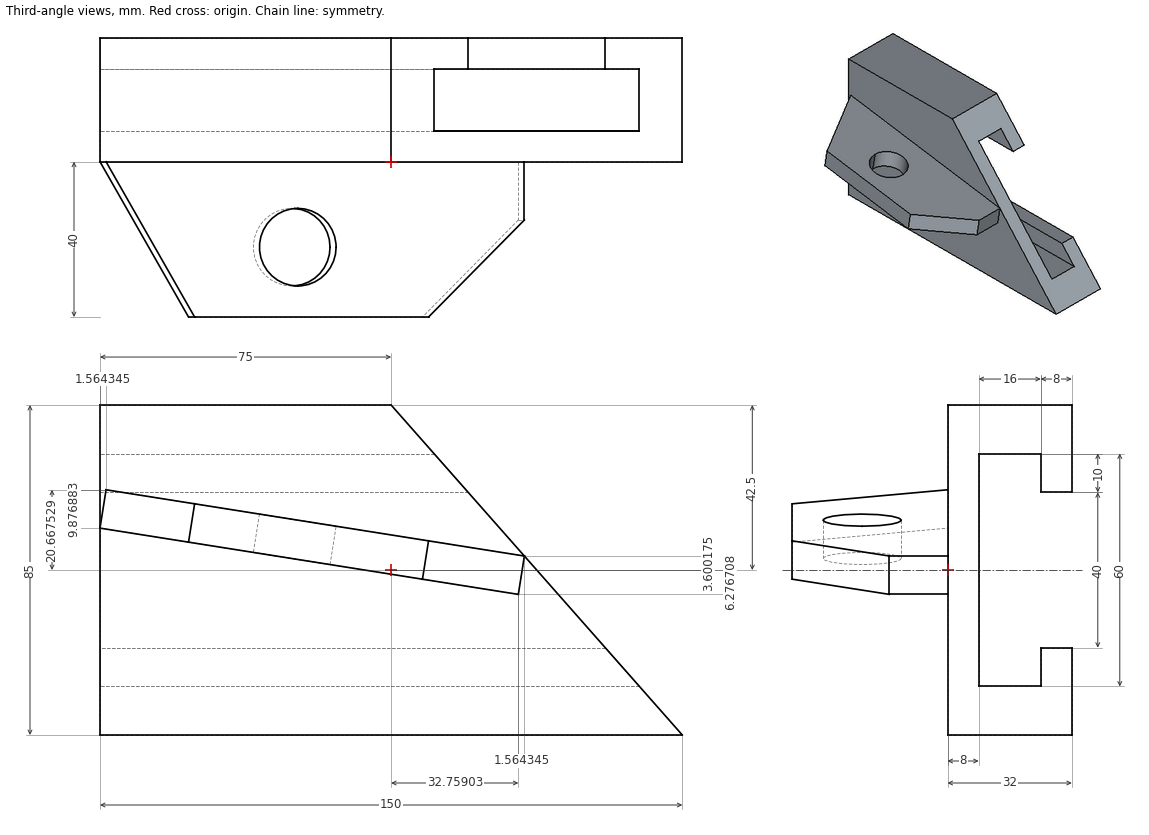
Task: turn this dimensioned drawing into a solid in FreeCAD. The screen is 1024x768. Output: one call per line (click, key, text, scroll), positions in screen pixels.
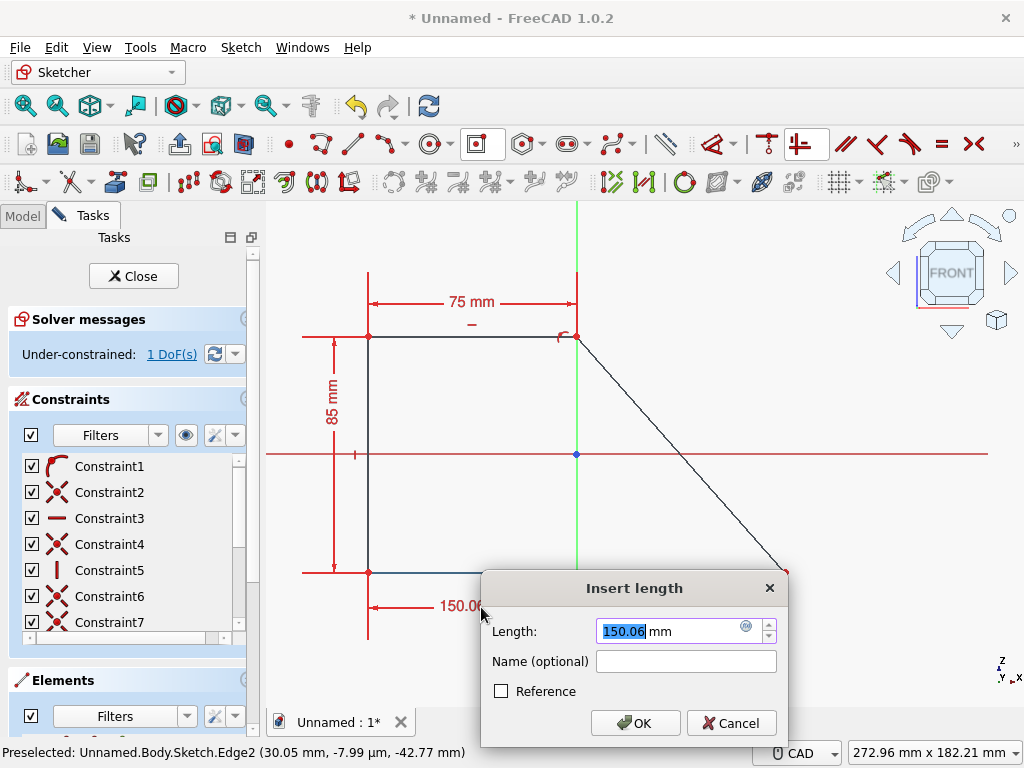
text(150)
key(Return)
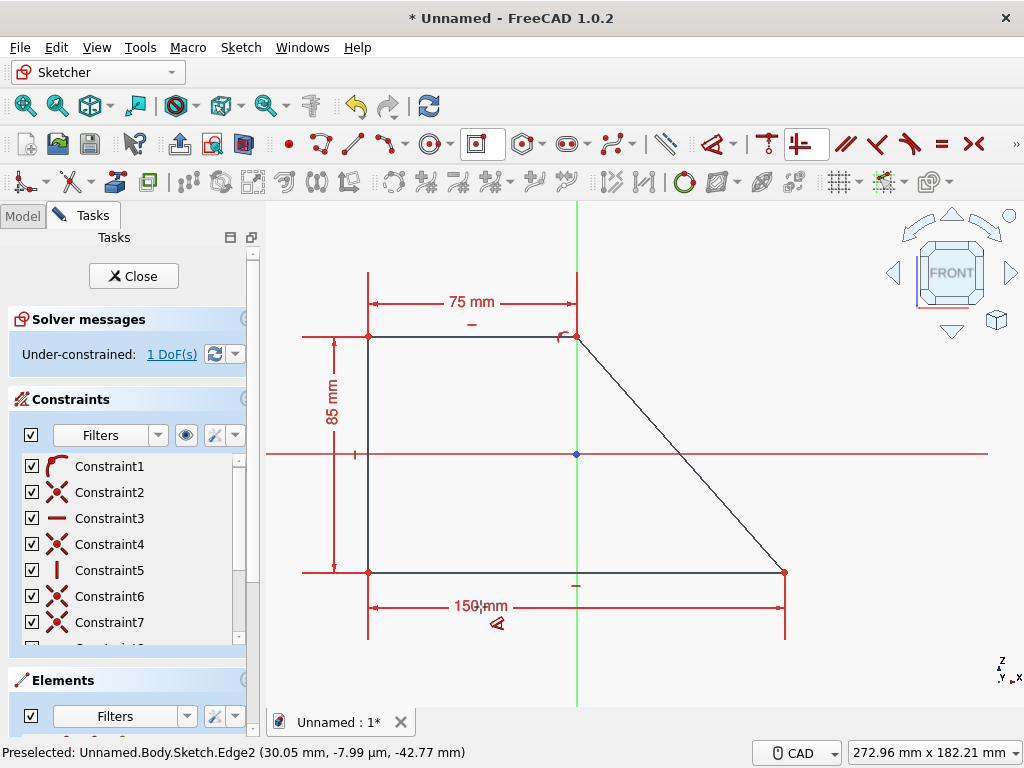
click(577, 337)
click(611, 396)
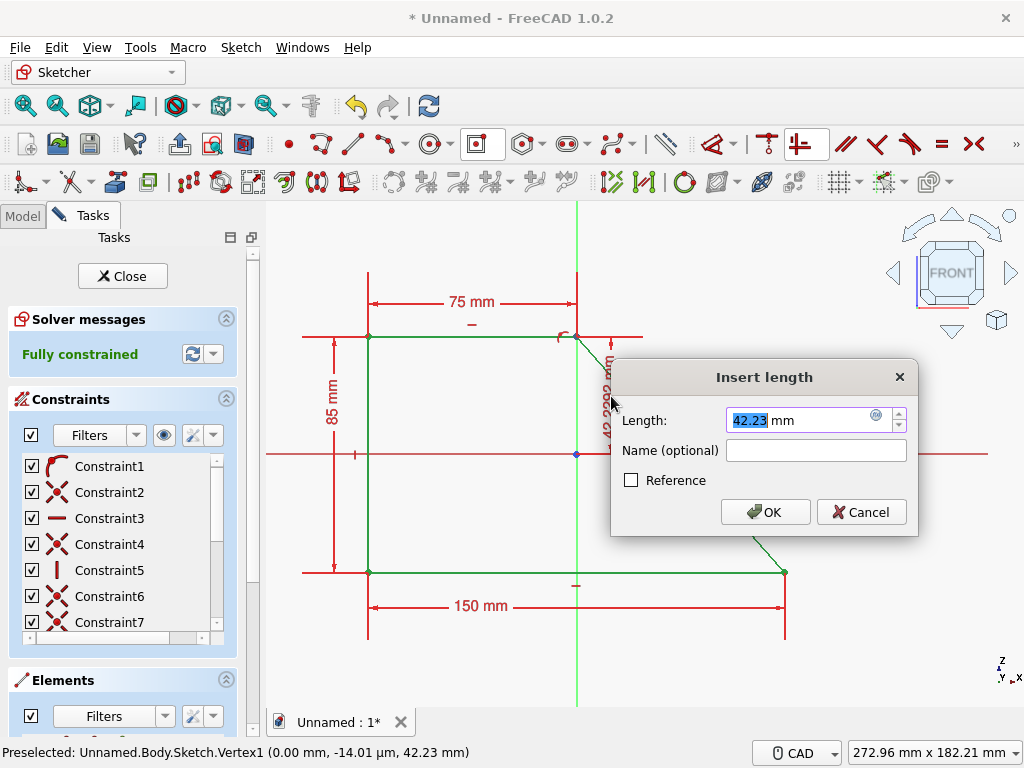
text(42.5)
key(Return)
key(Escape)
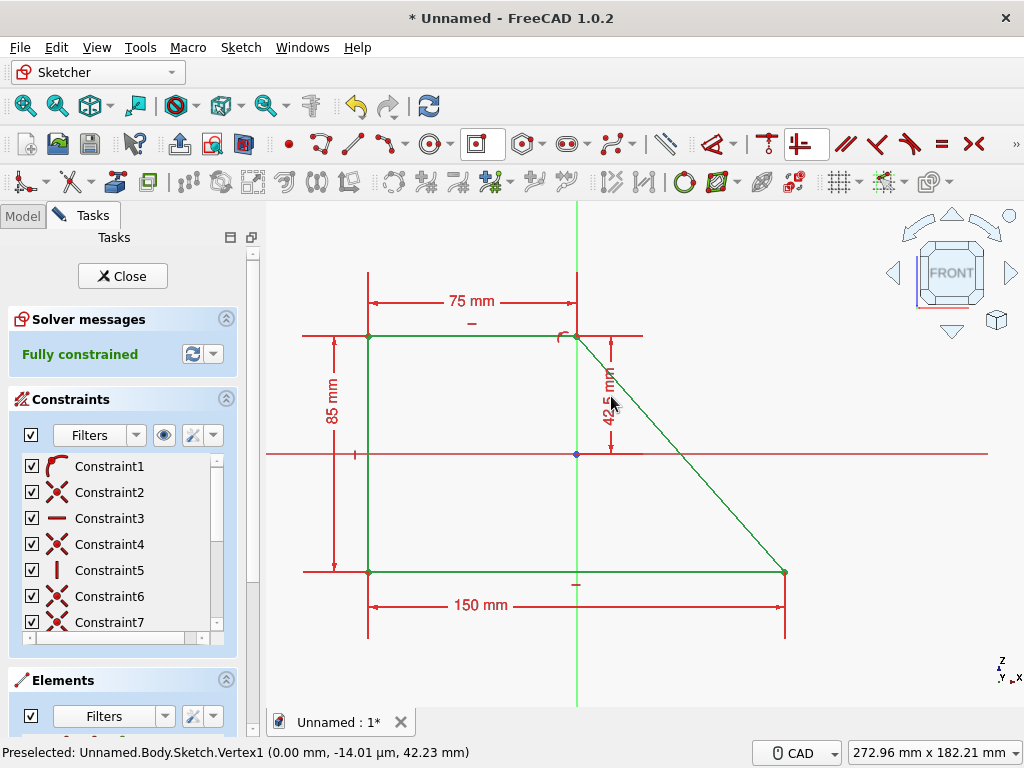
click(123, 276)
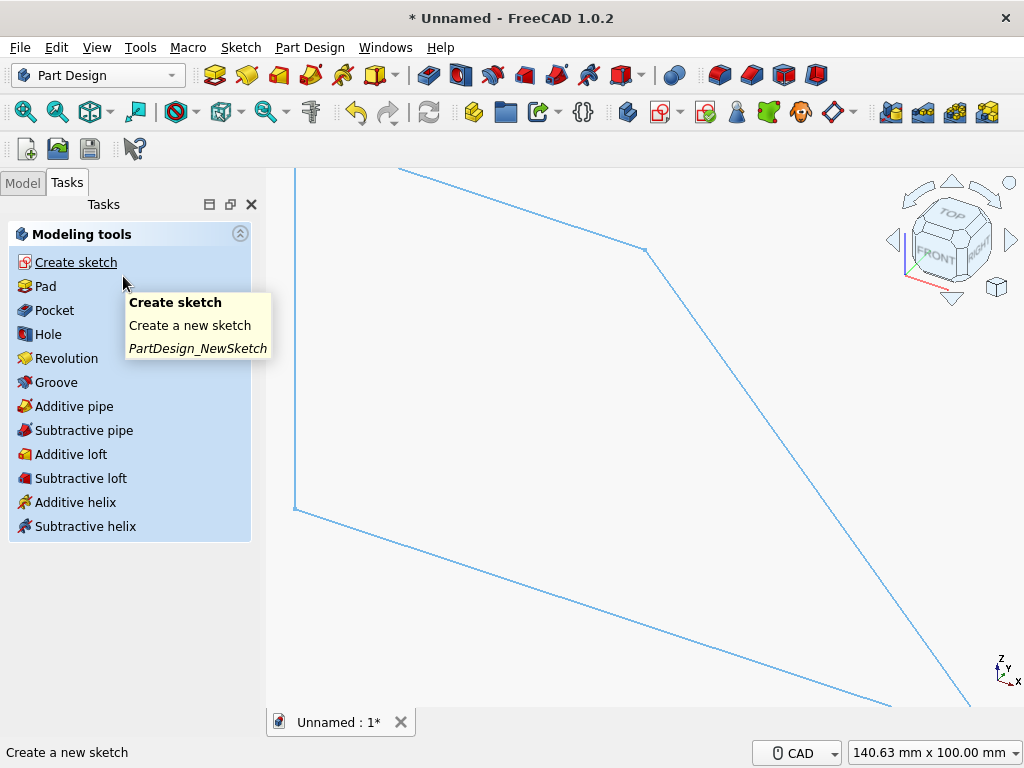
click(216, 76)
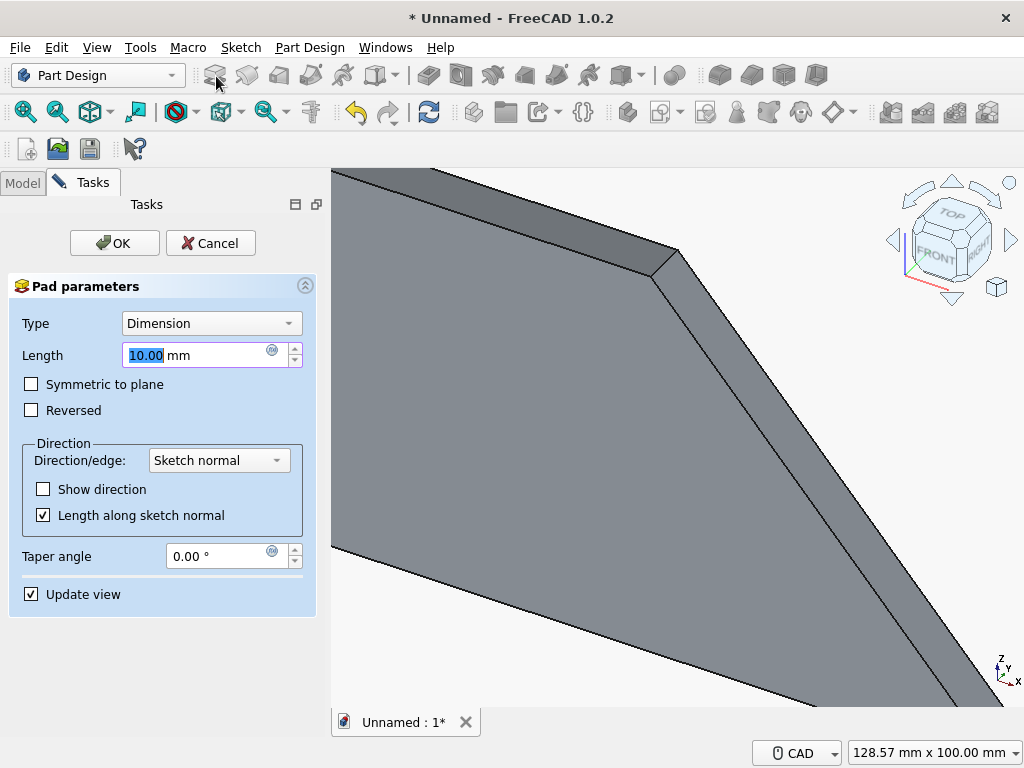
text(32)
key(Tab)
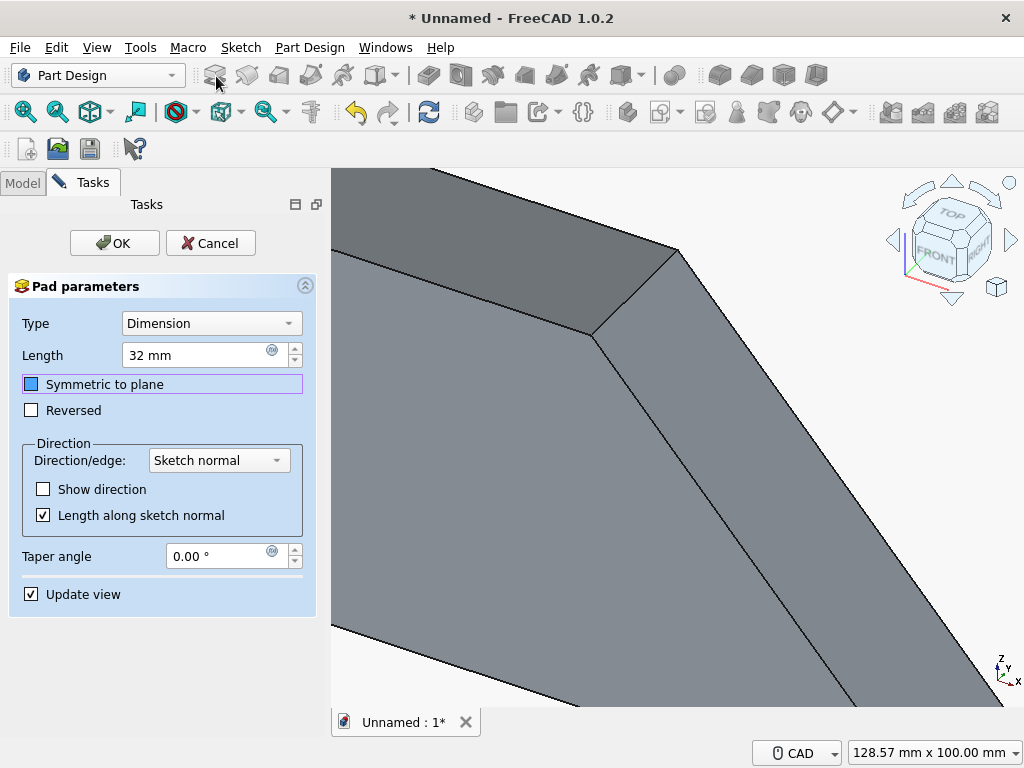
click(30, 410)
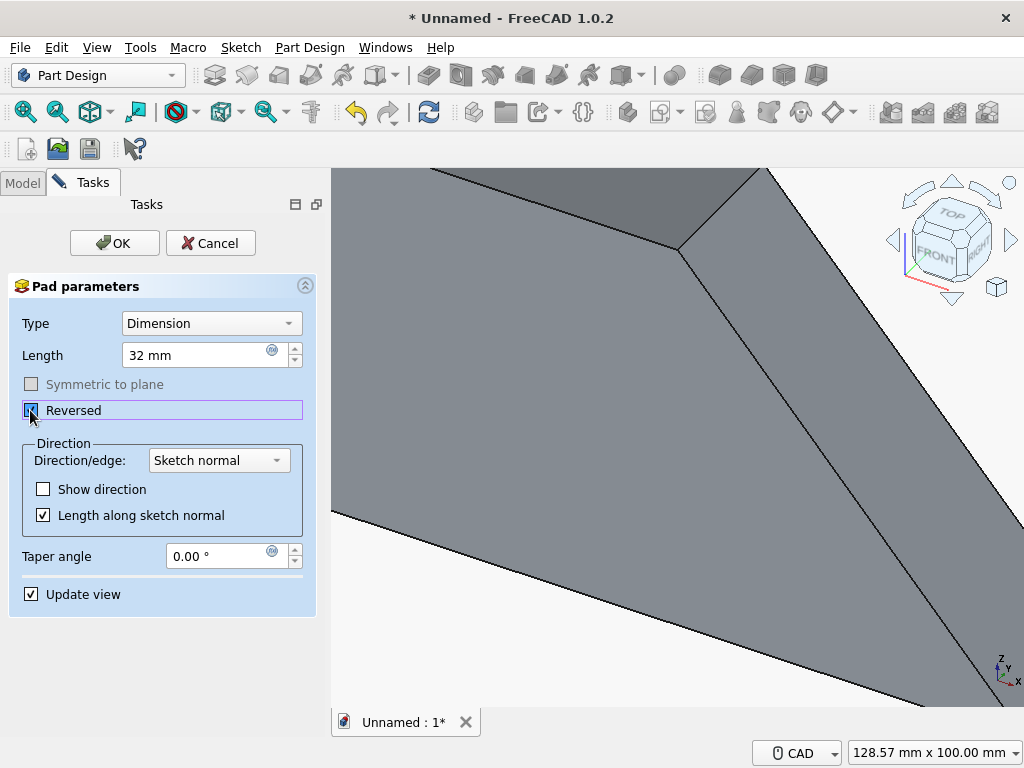
click(115, 243)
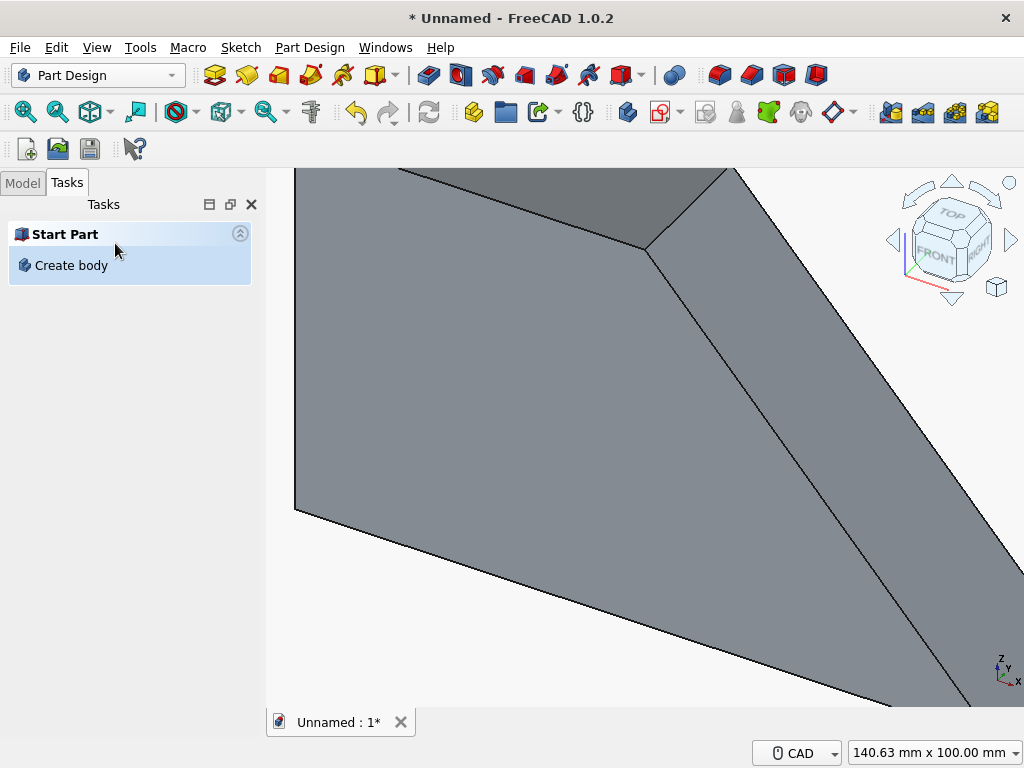
key(v)
key(f)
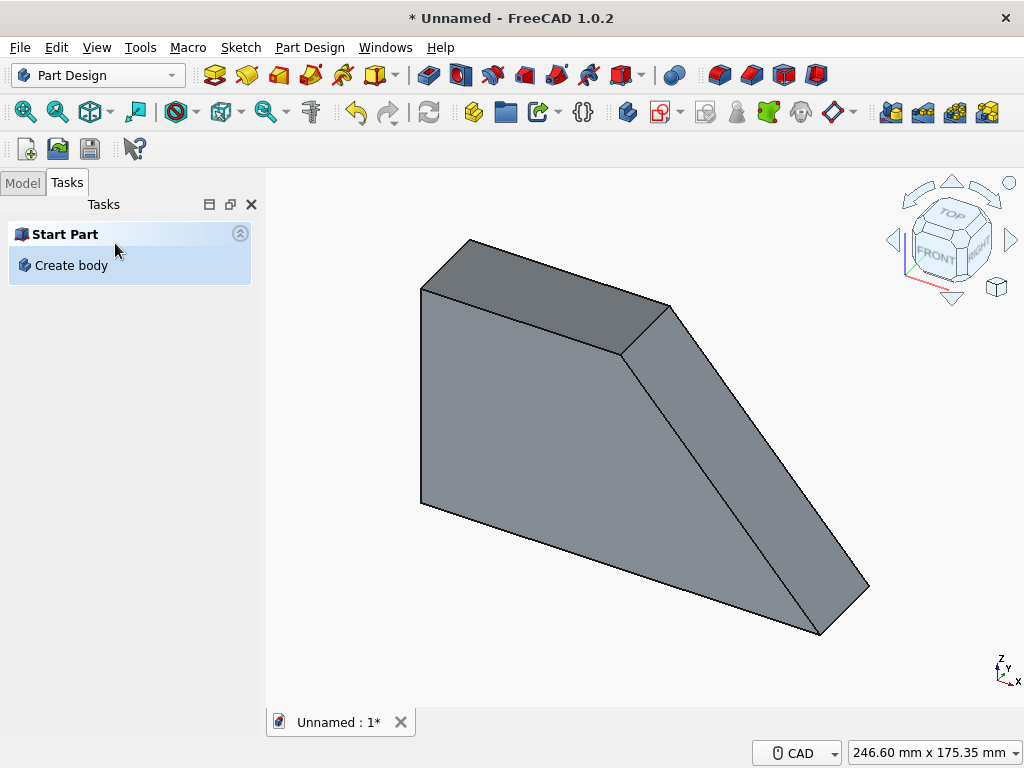
key(6)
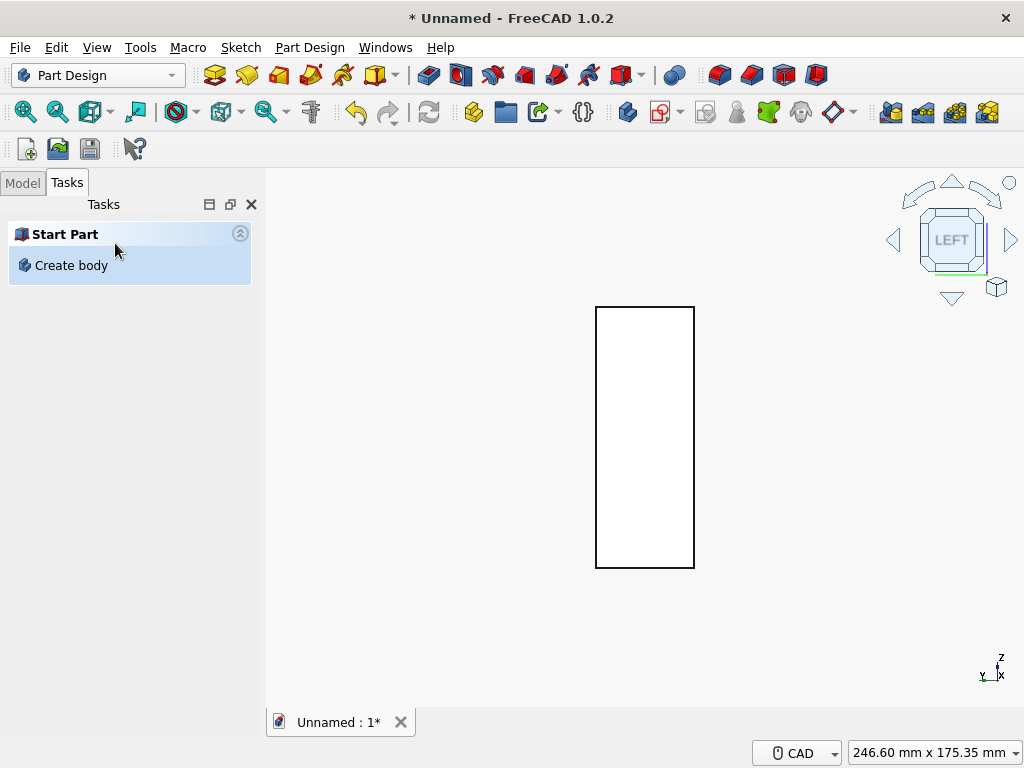
click(645, 511)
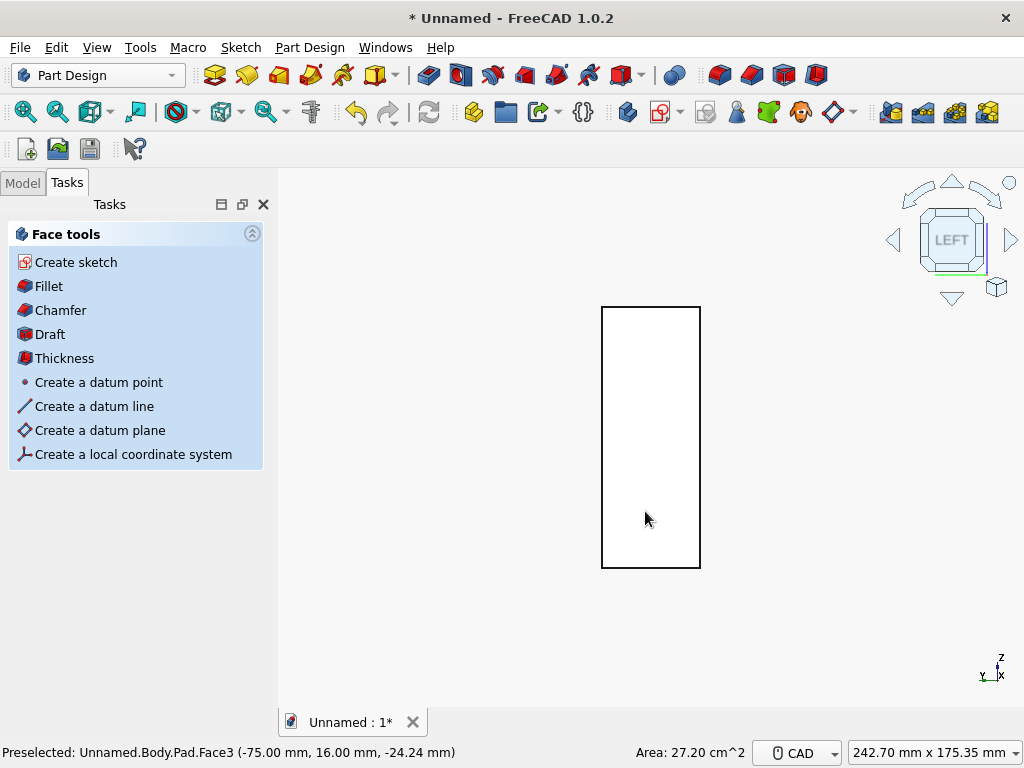
click(660, 112)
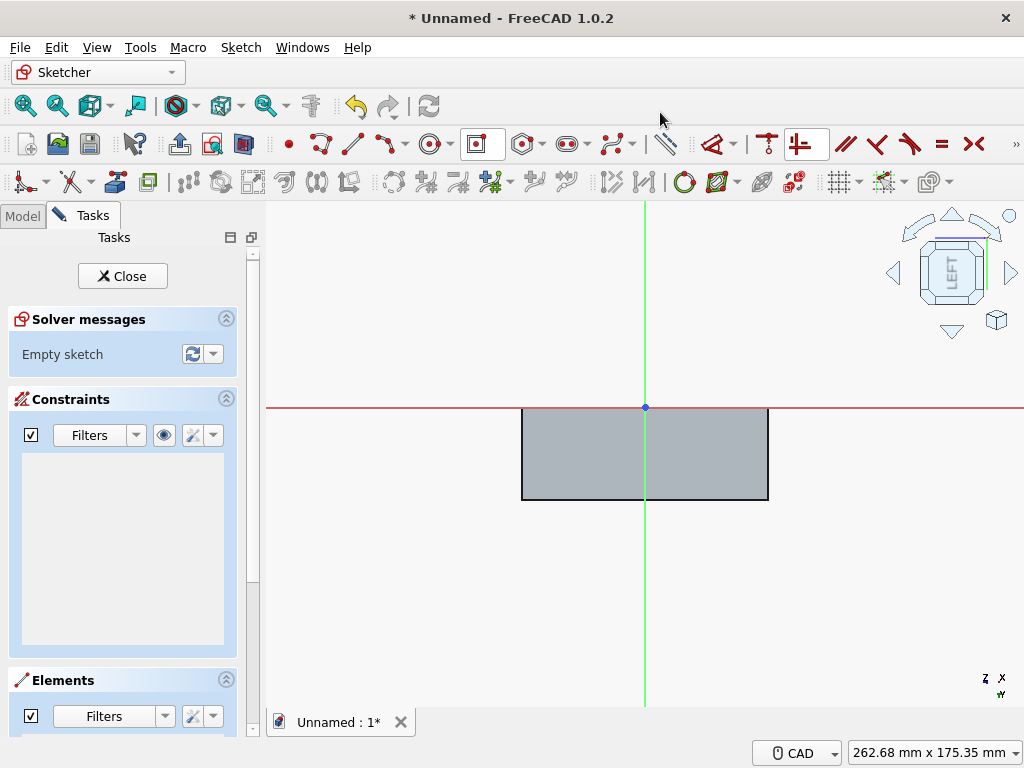
scroll(701, 454, up, 4)